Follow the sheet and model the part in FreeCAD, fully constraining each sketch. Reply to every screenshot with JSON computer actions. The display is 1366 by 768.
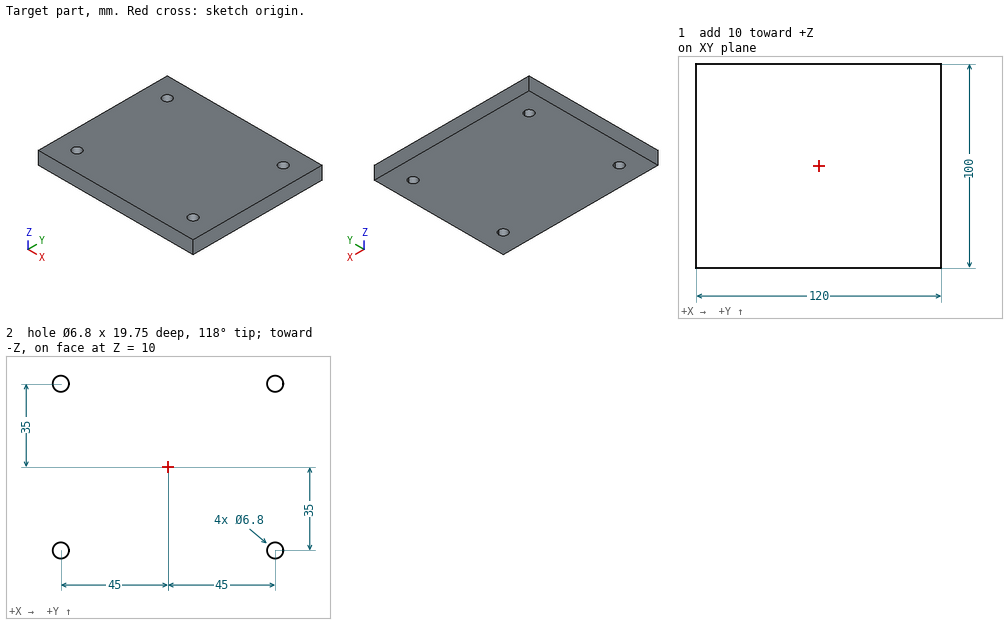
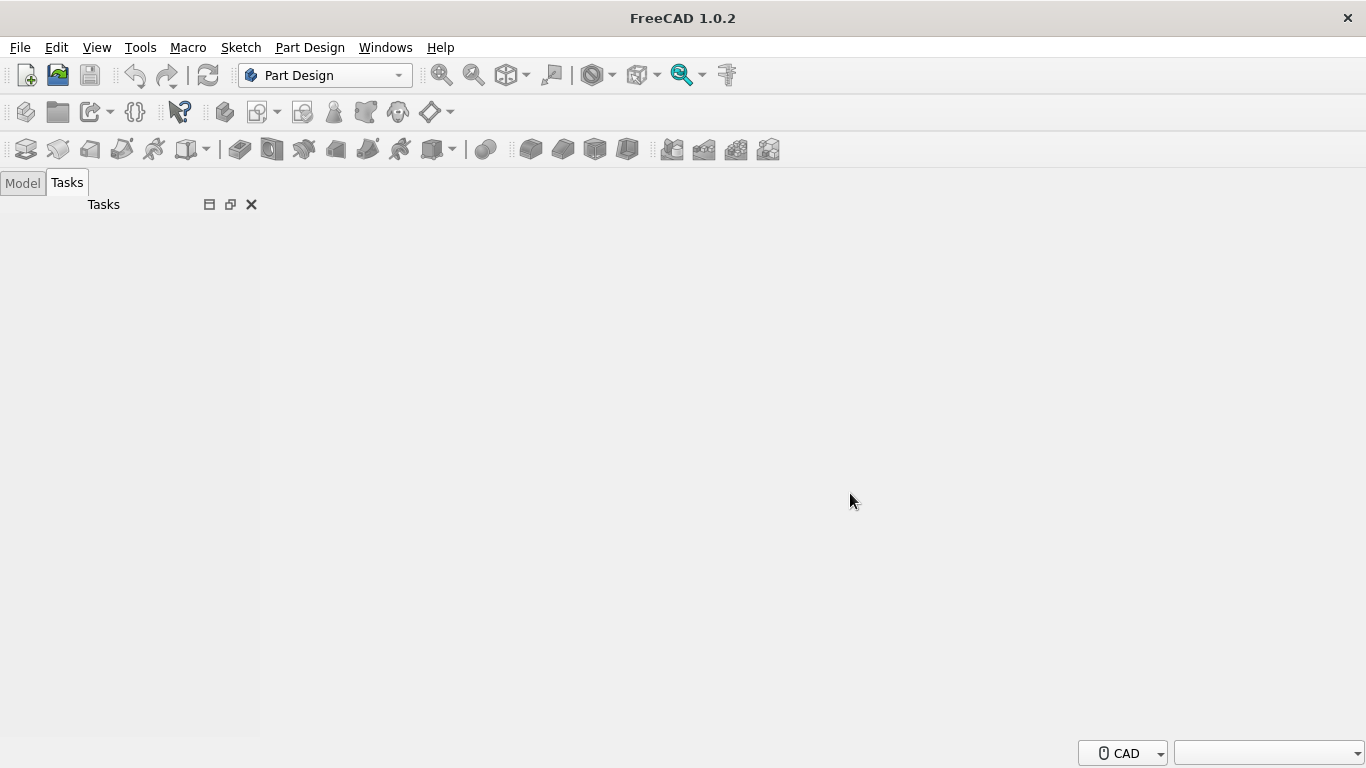
{"action": "key", "text": "ctrl+n"}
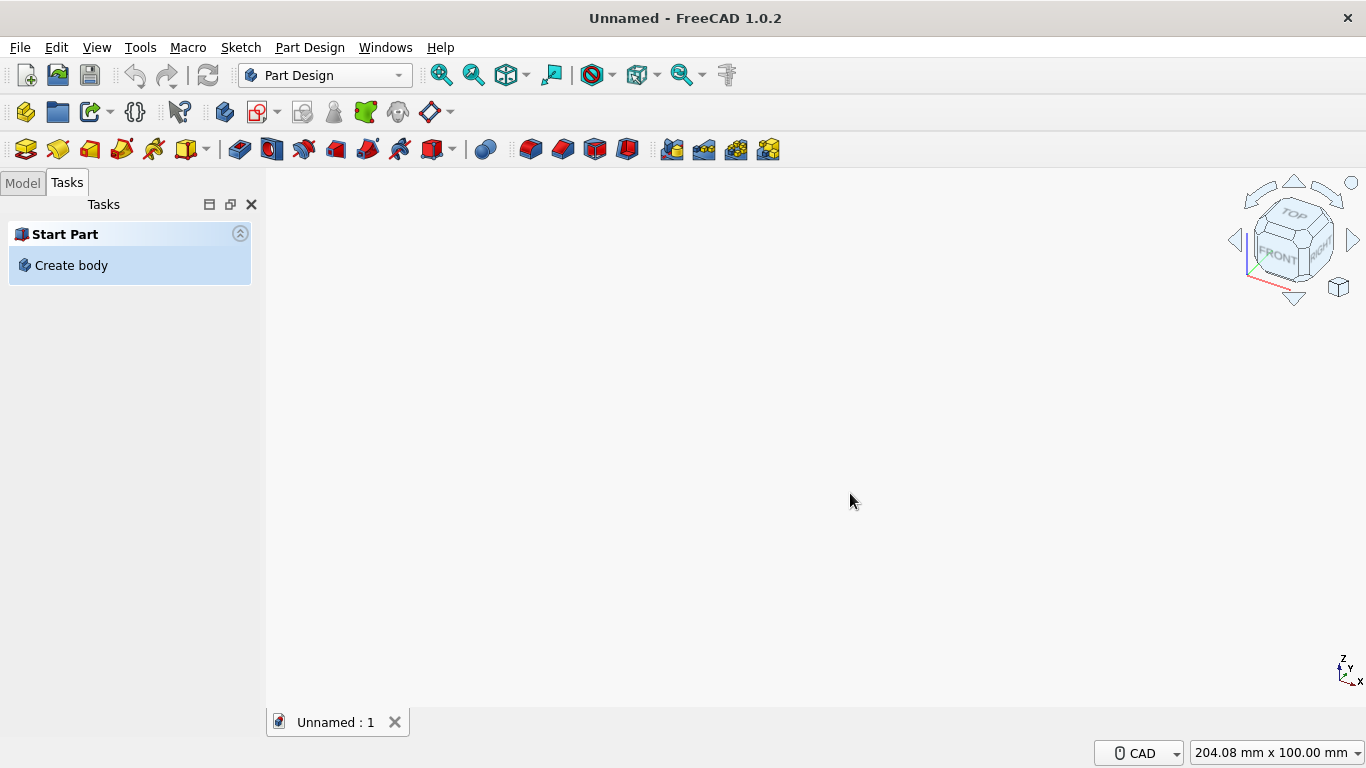
{"action": "left_click", "coordinate": [258, 112]}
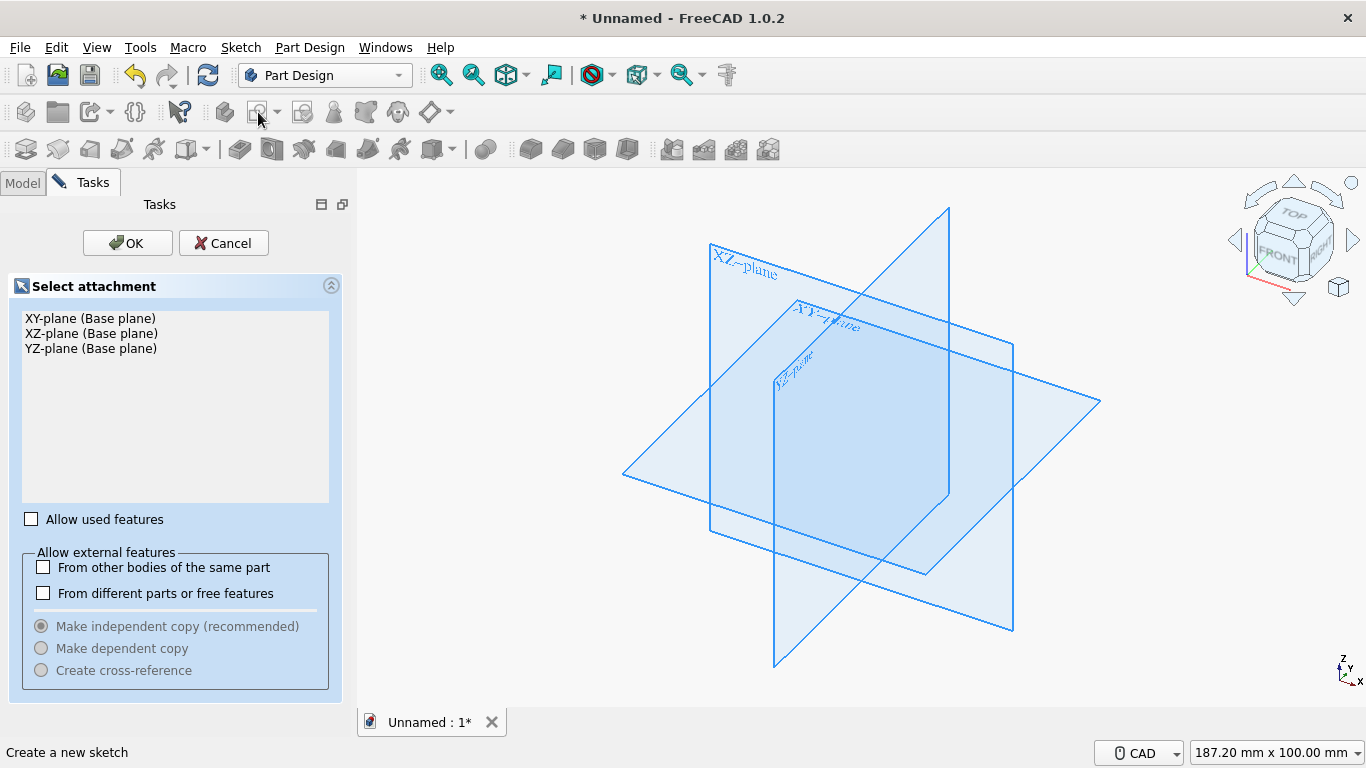
{"action": "left_click", "coordinate": [82, 318]}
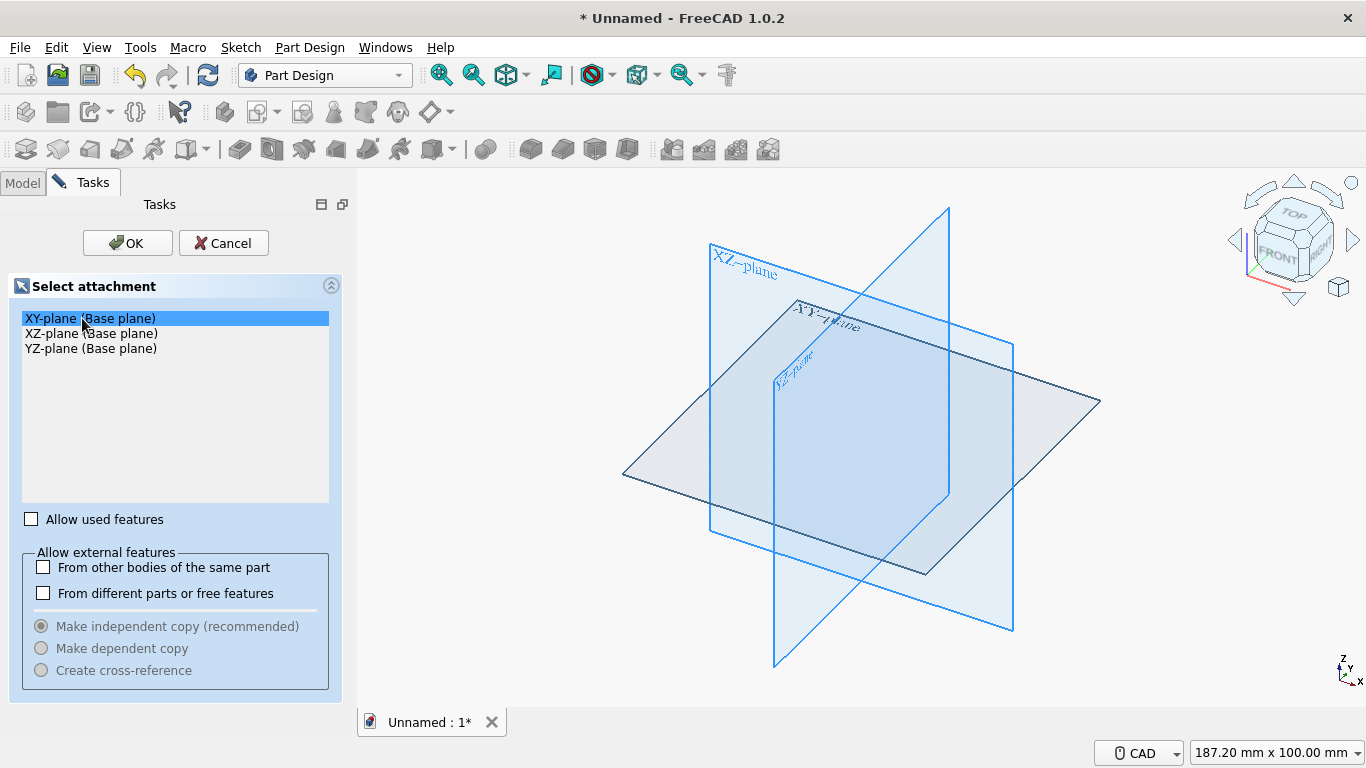
{"action": "left_click", "coordinate": [128, 243]}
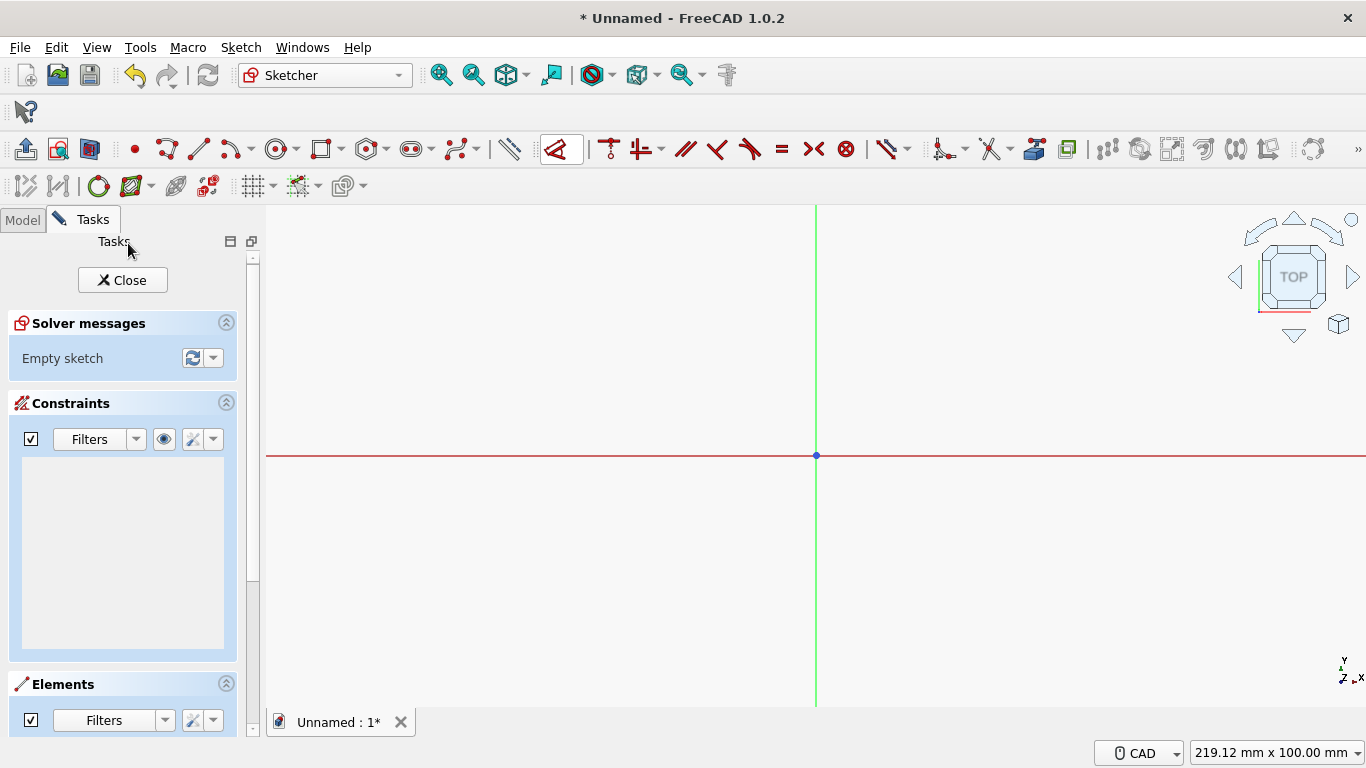
{"action": "scroll", "coordinate": [608, 456], "scroll_direction": "down", "scroll_amount": 2}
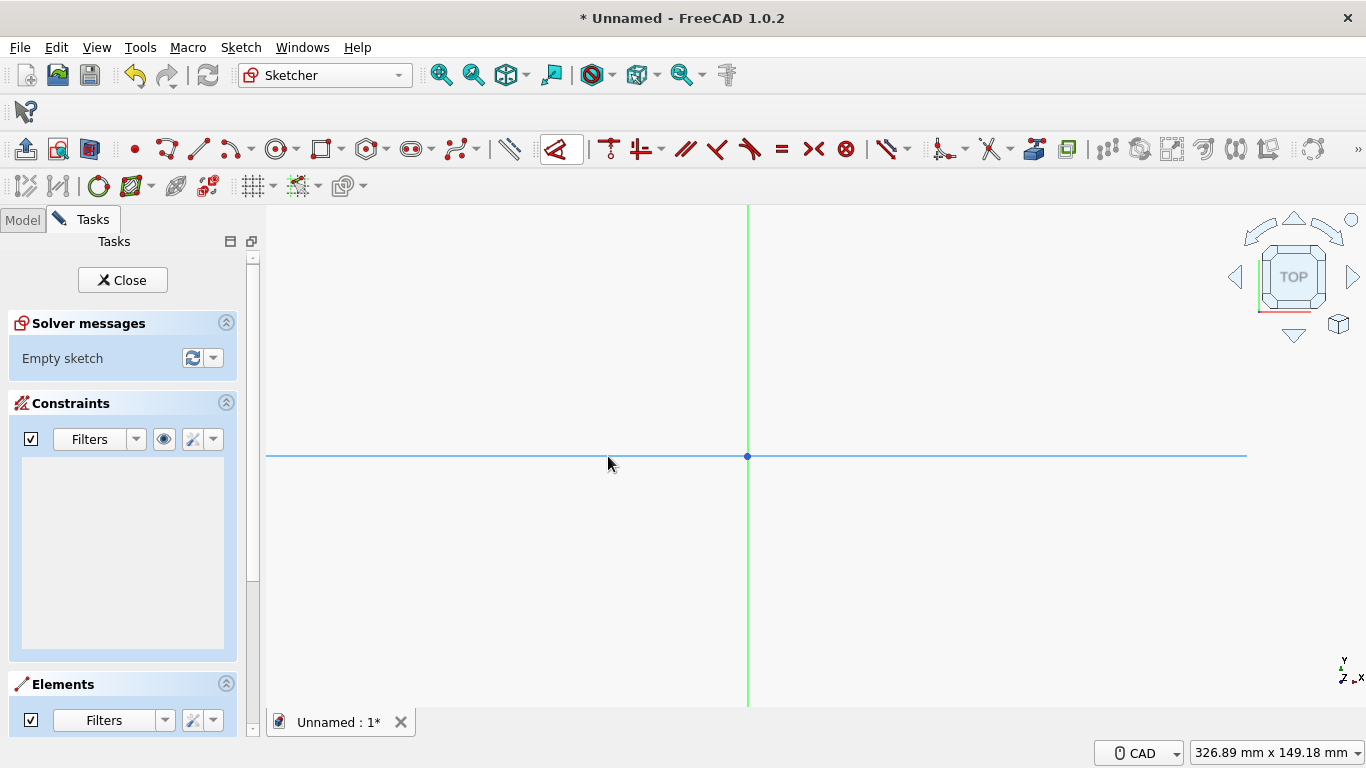
{"action": "left_click", "coordinate": [344, 150]}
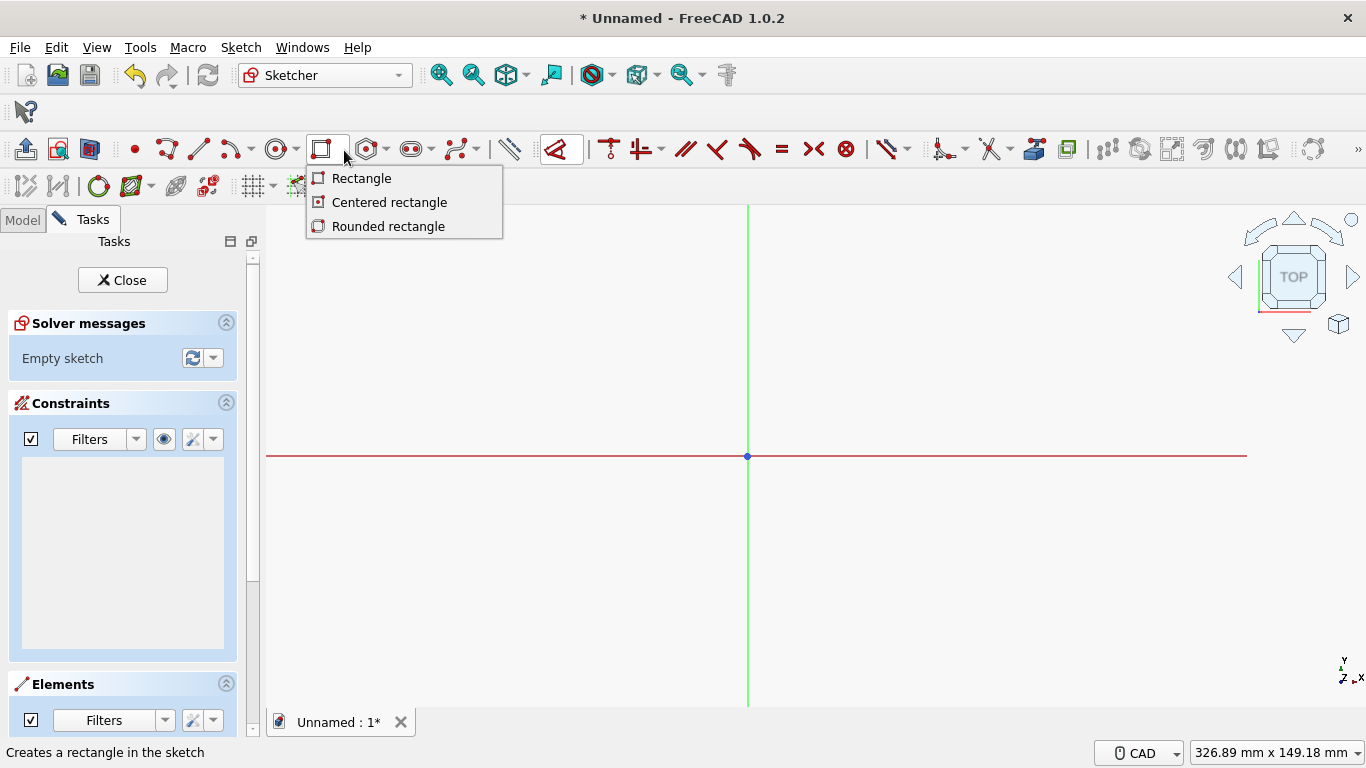
{"action": "left_click", "coordinate": [404, 202]}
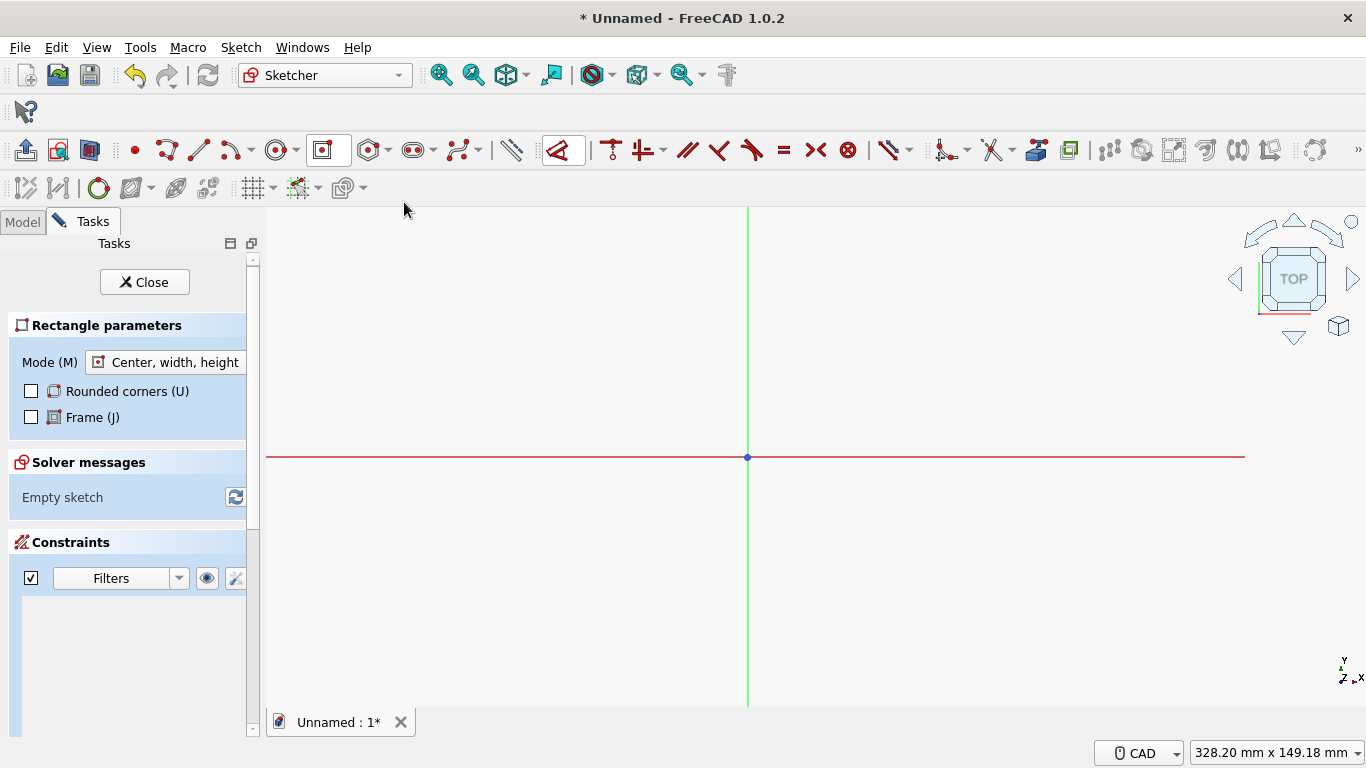
{"action": "left_click", "coordinate": [748, 457]}
{"action": "left_click", "coordinate": [949, 290]}
{"action": "key", "text": "Escape"}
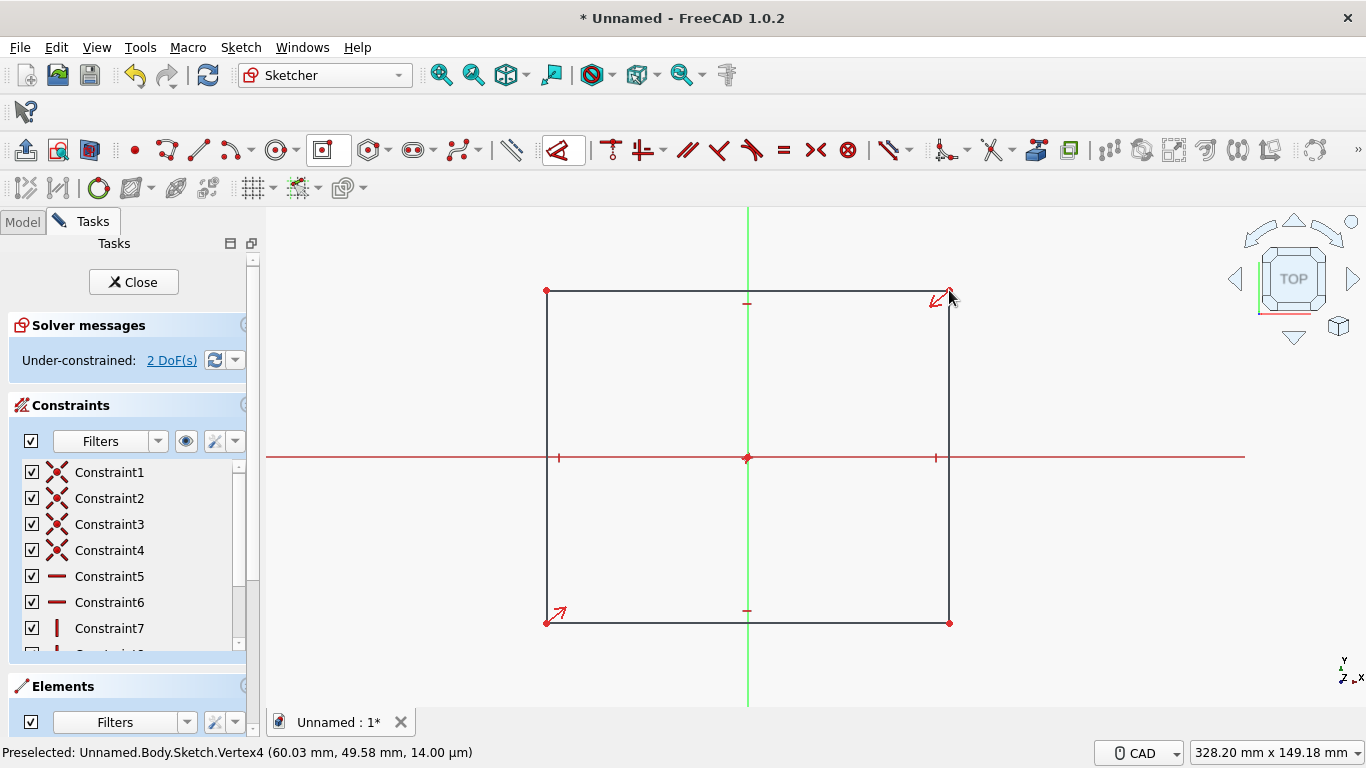
{"action": "left_click", "coordinate": [558, 150]}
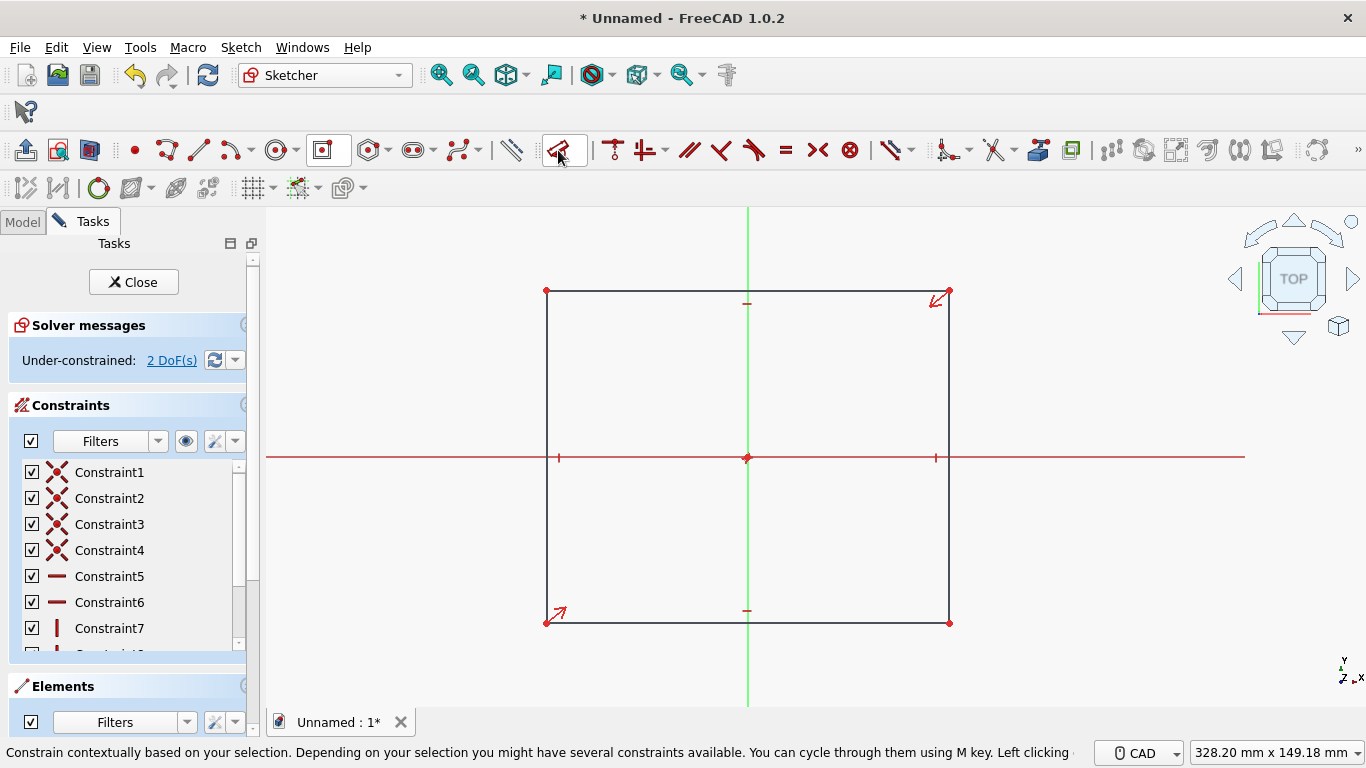
{"action": "left_click", "coordinate": [667, 623]}
{"action": "left_click", "coordinate": [655, 657]}